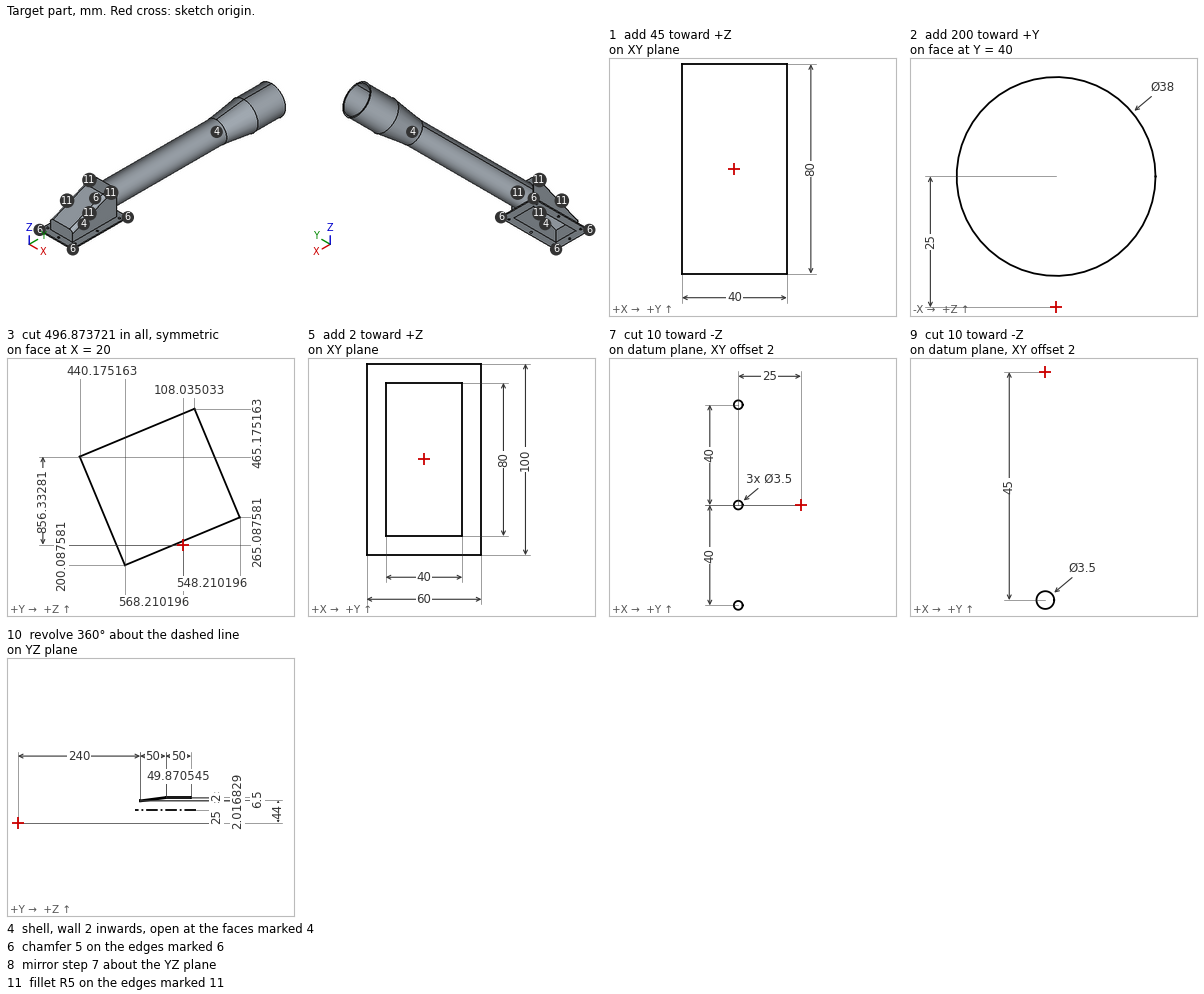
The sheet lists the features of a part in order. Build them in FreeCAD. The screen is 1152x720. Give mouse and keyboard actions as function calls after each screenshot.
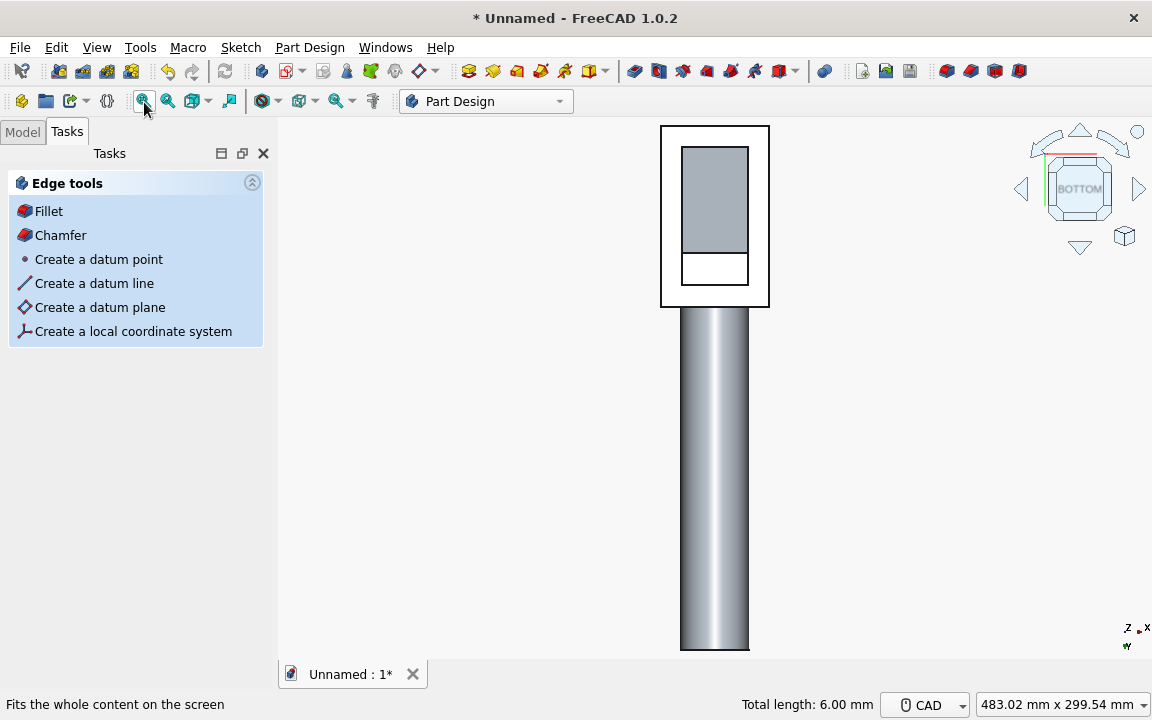
click(144, 102)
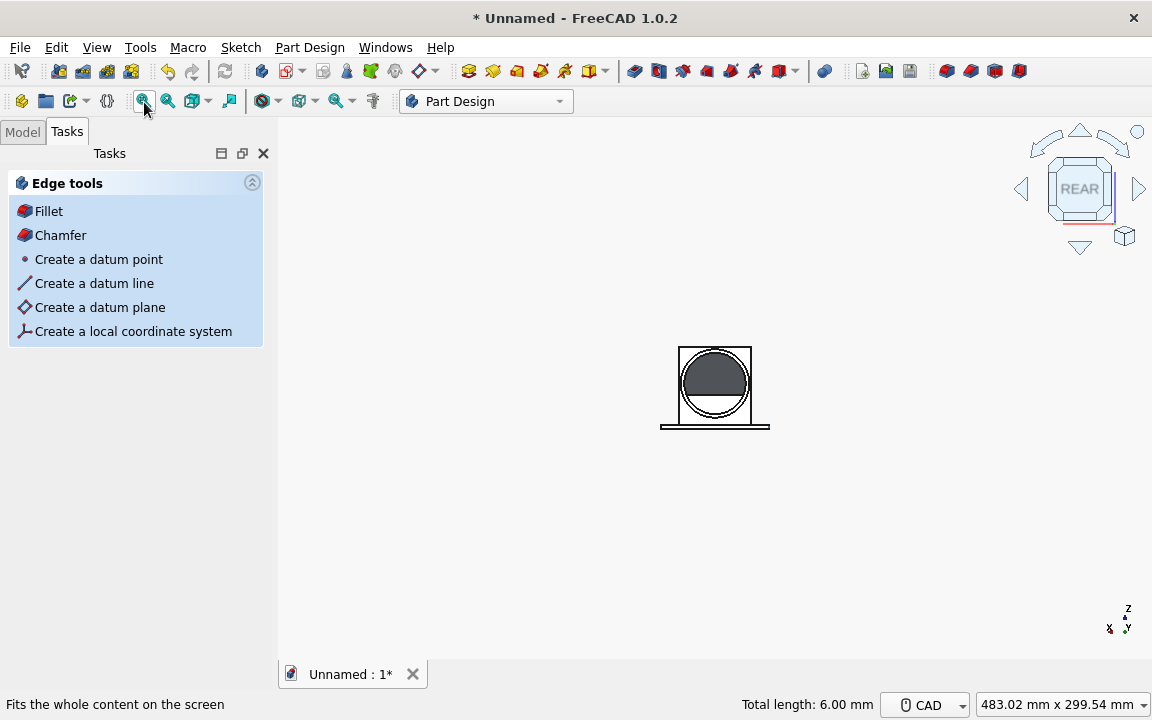
scroll(661, 426, up, 13)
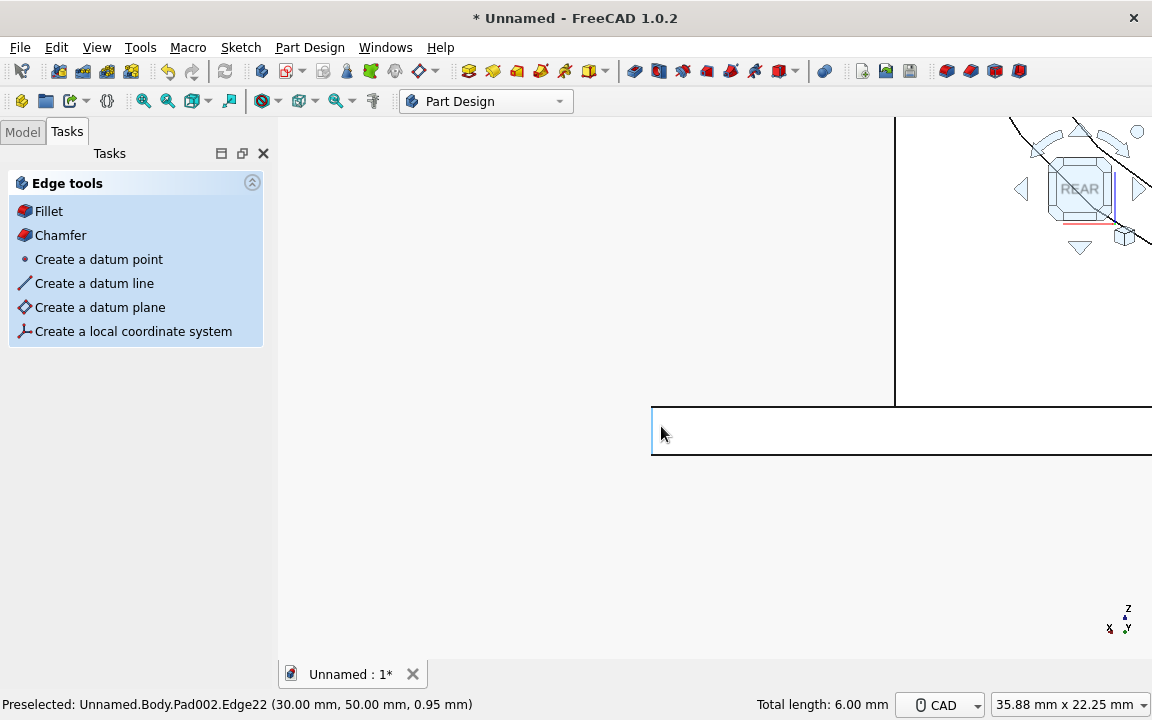
click(652, 430, ctrl)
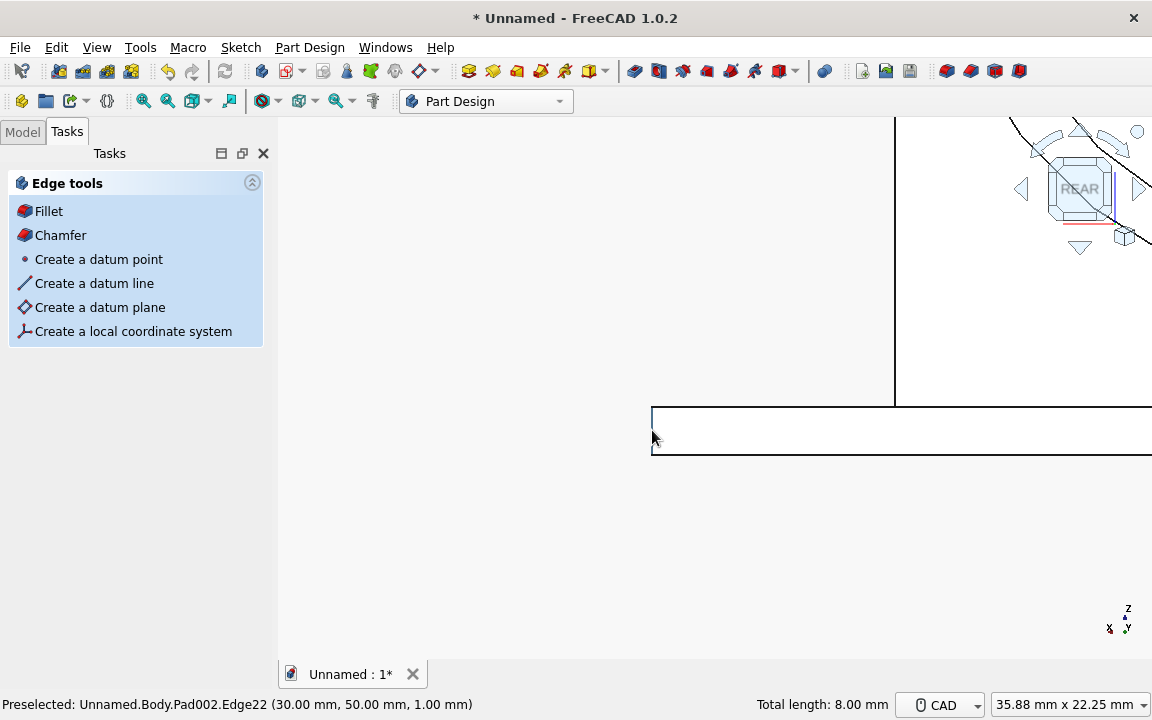
click(972, 72)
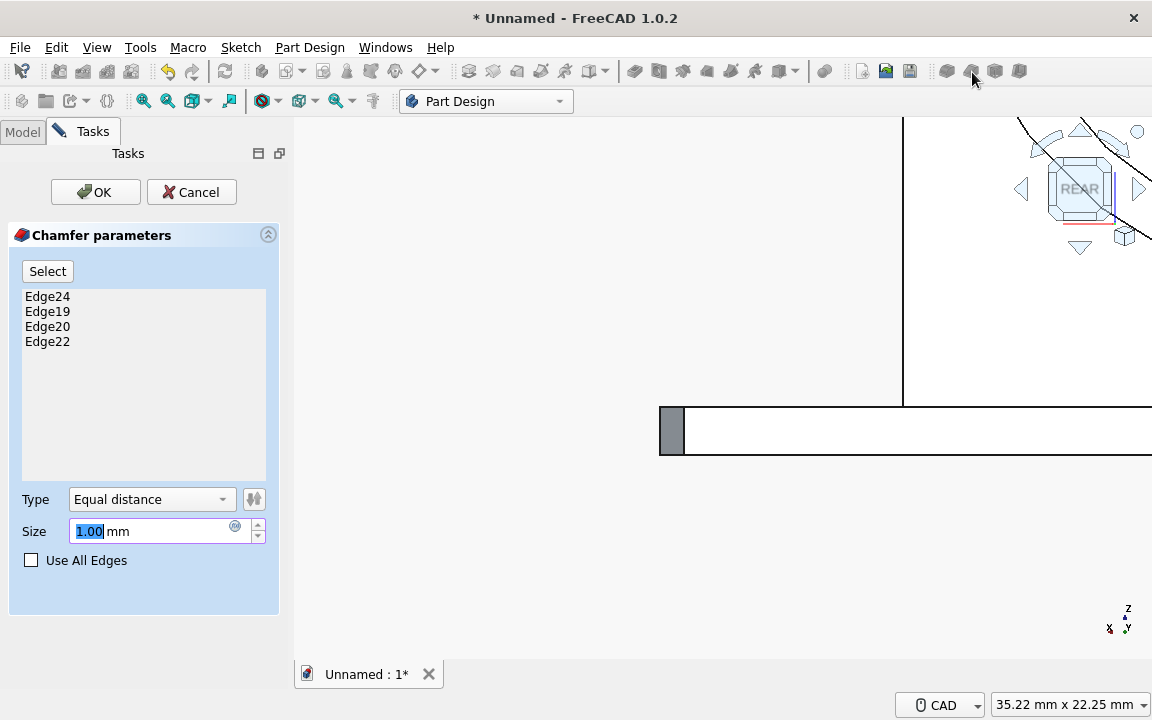
text(5)
key(Tab)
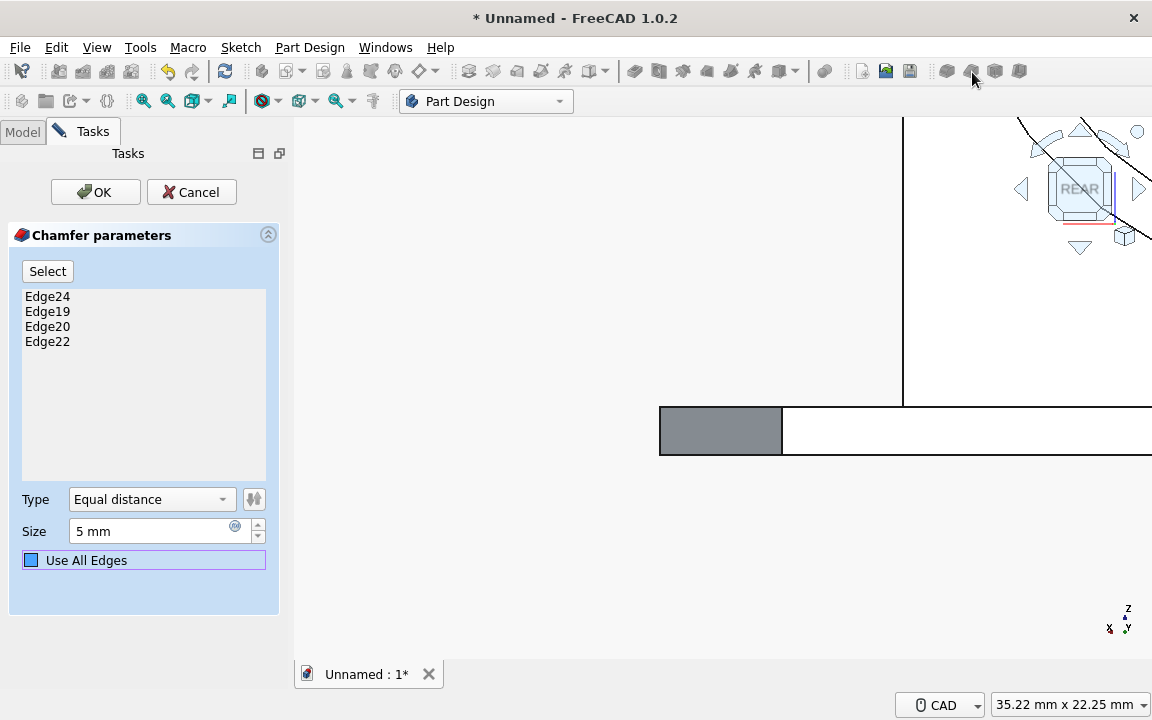
click(96, 192)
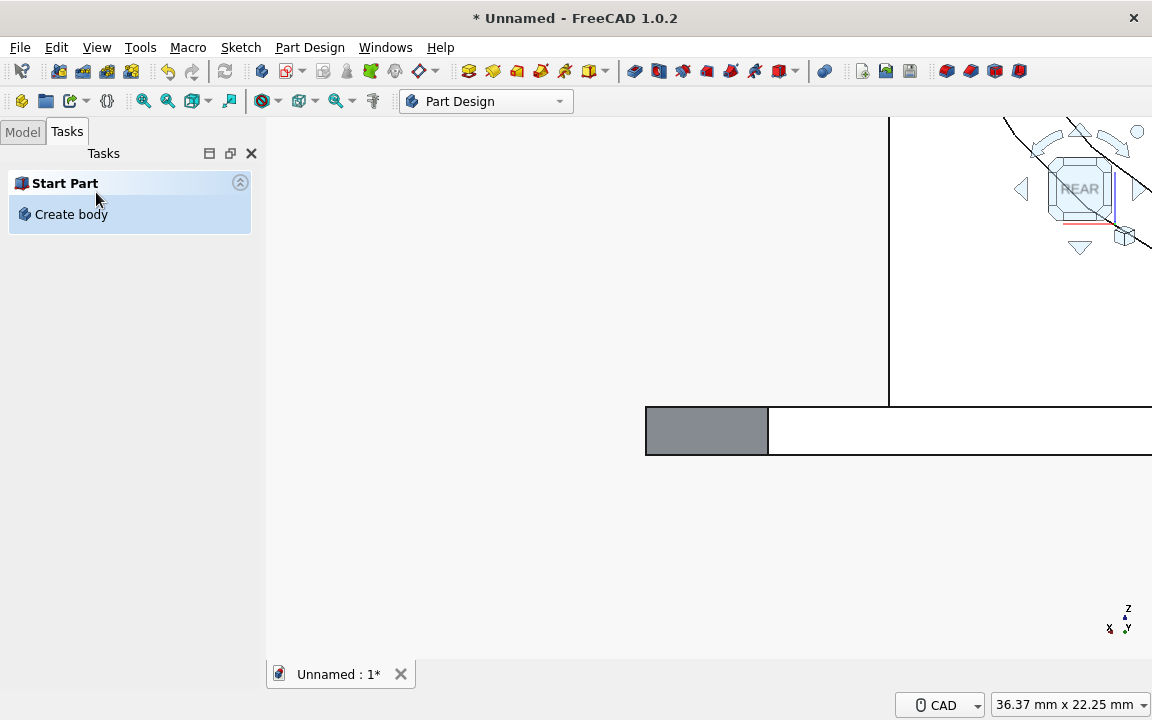
key(v)
key(f)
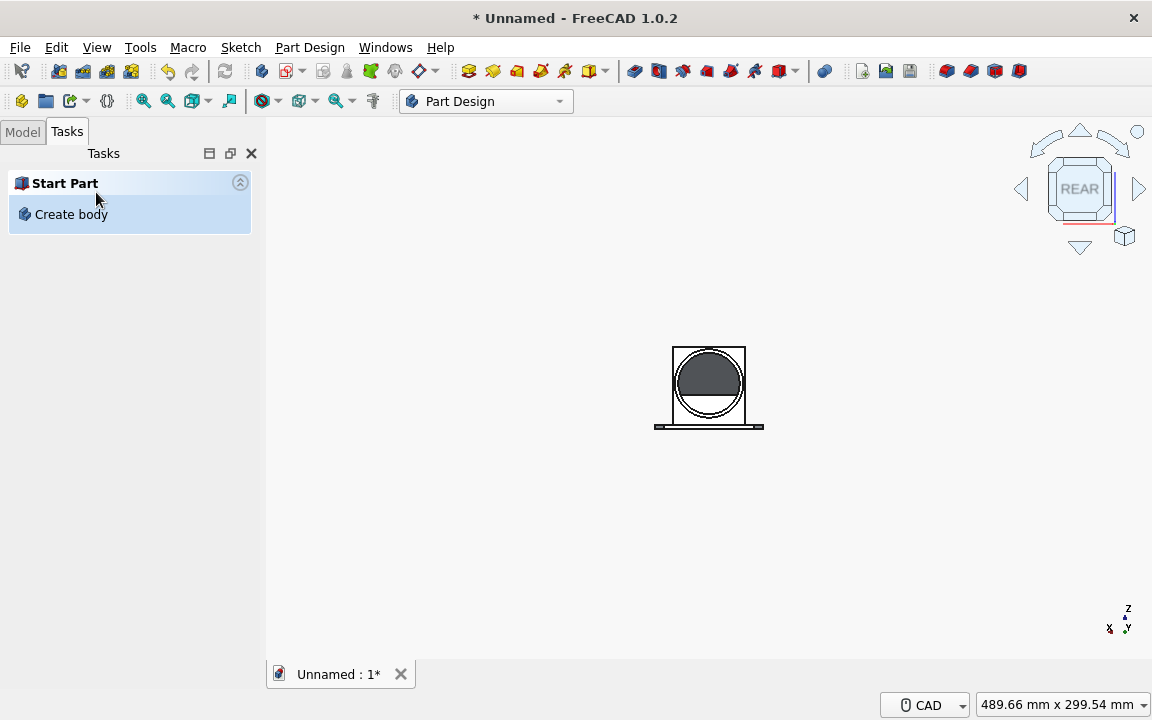
key(0)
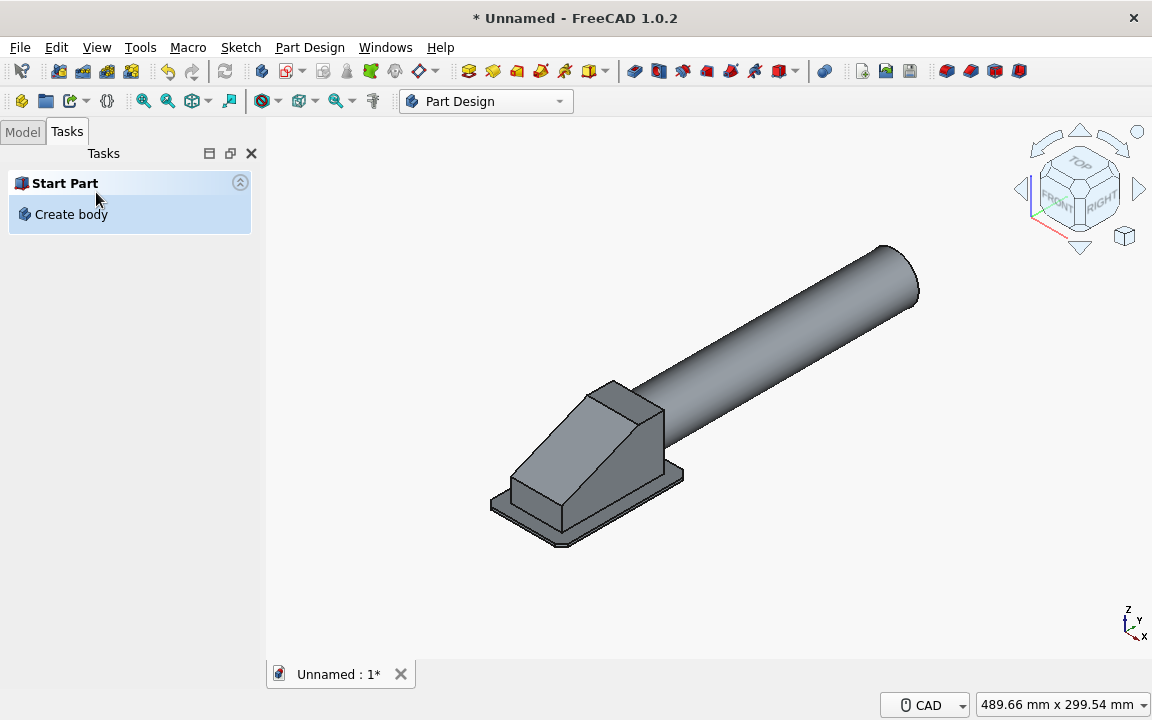
key(2)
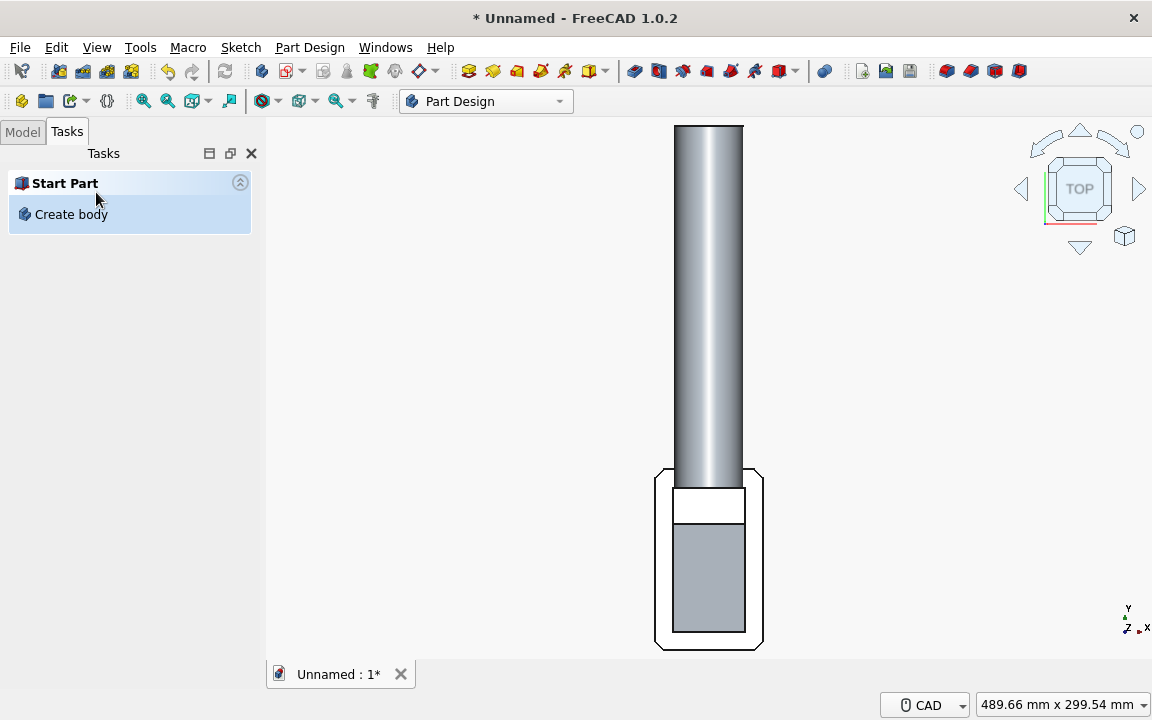
key(1)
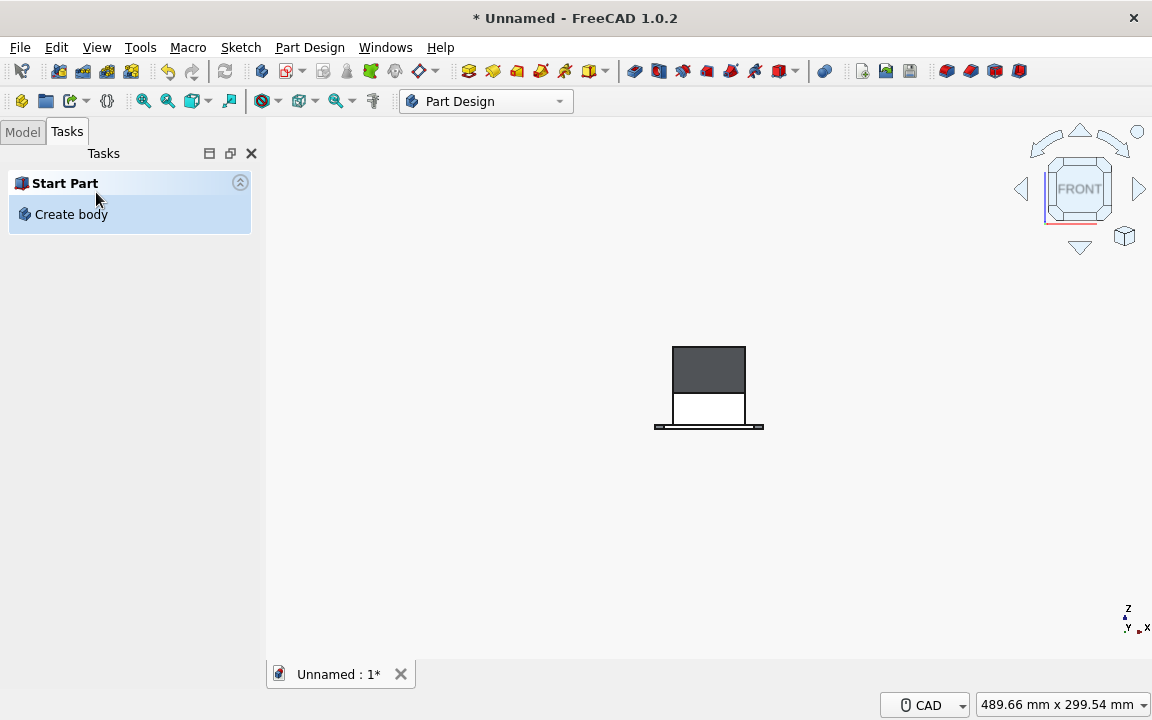
key(v)
key(f)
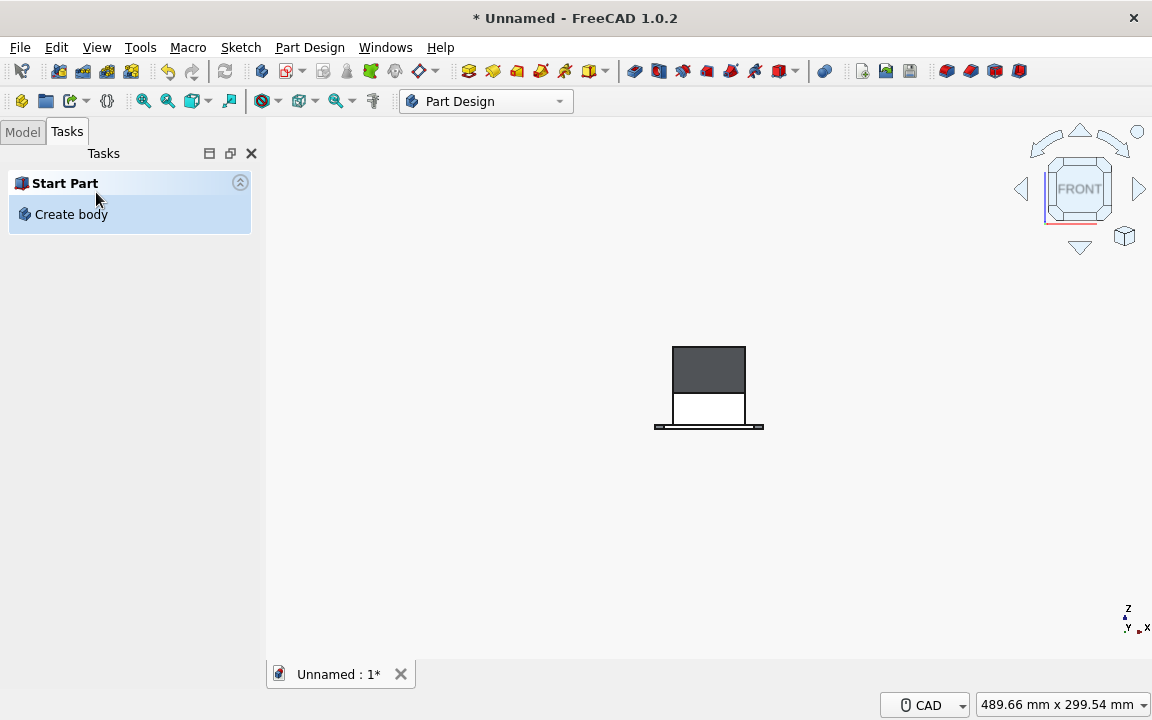
click(23, 131)